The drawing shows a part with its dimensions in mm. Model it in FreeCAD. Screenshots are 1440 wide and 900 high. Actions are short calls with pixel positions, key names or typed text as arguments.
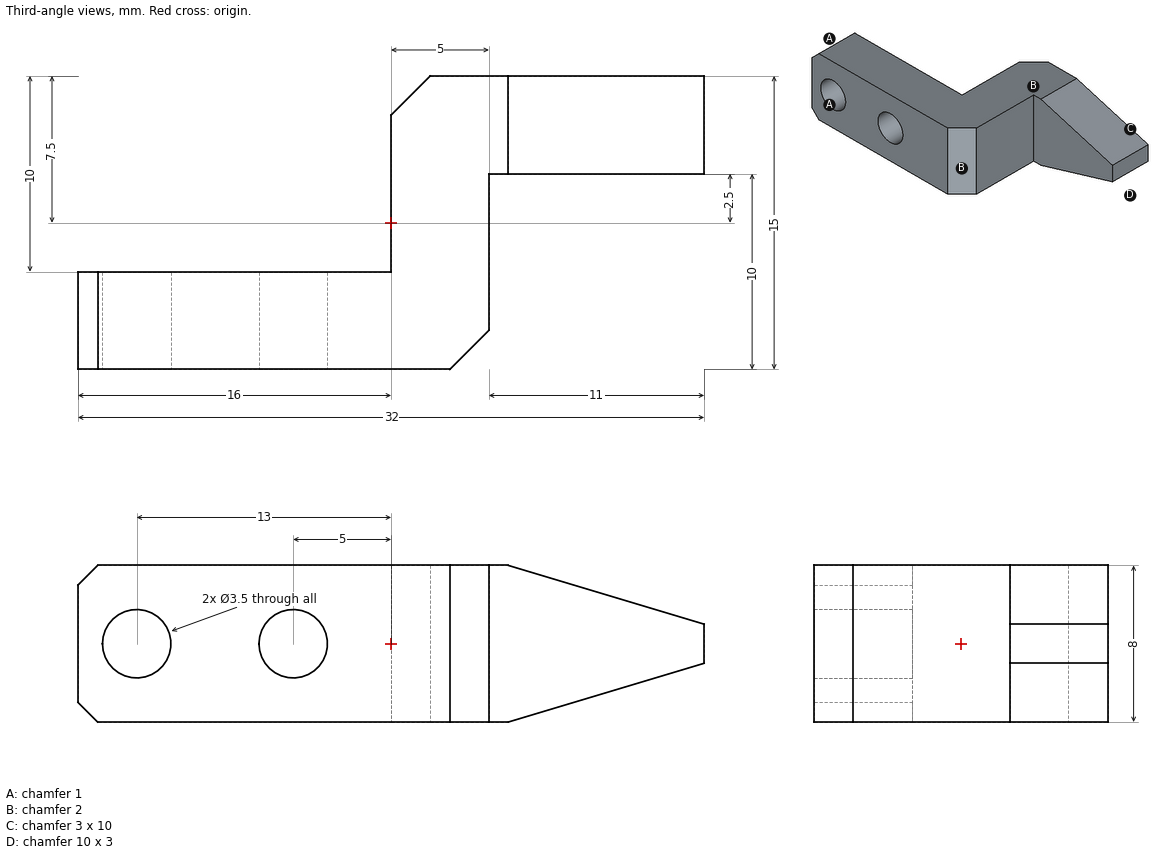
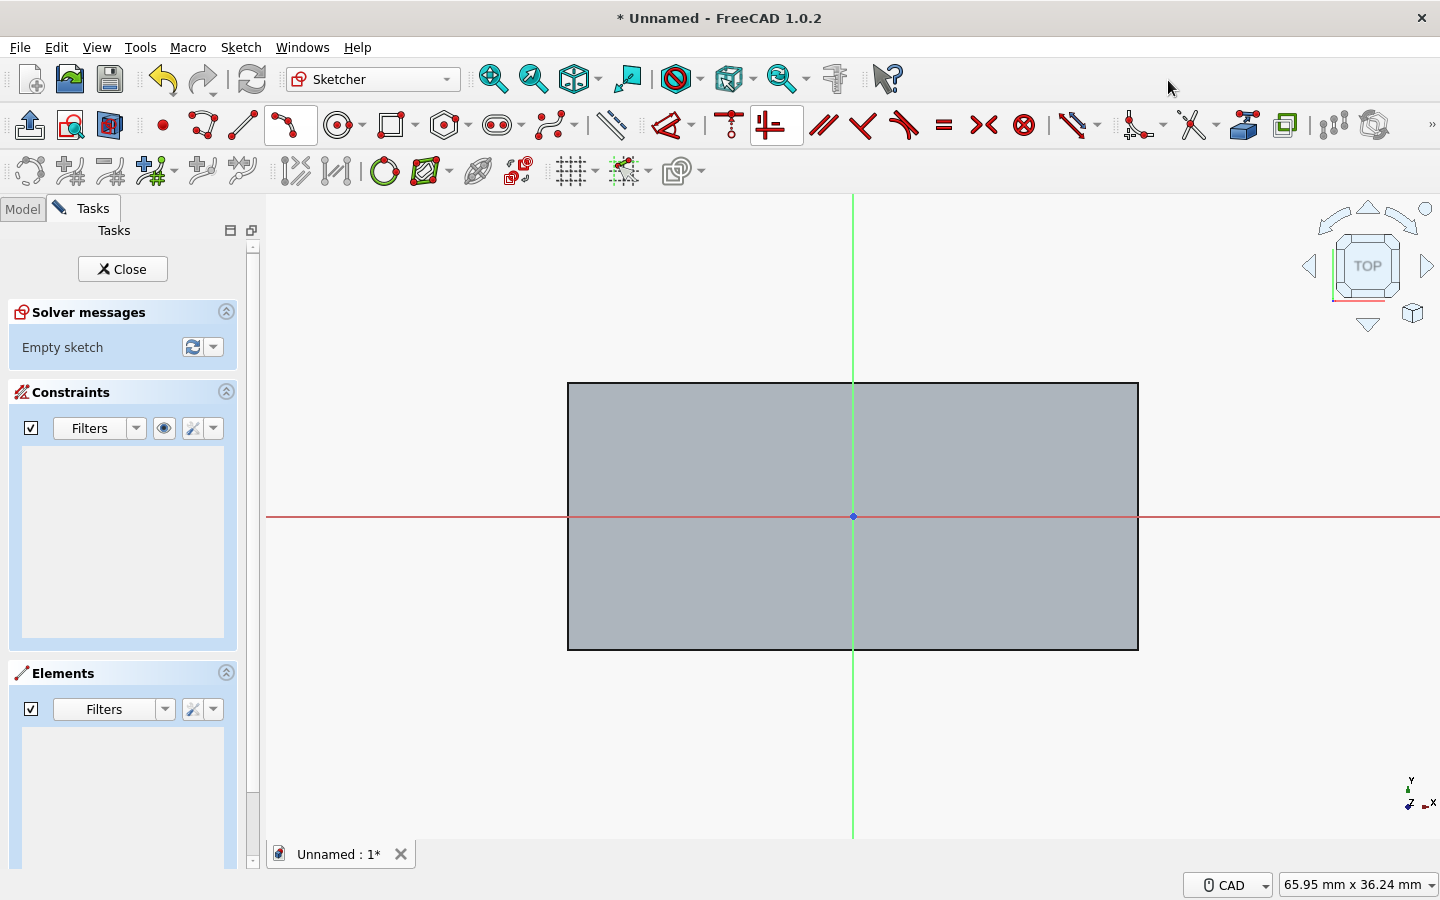
key(g)
key(r)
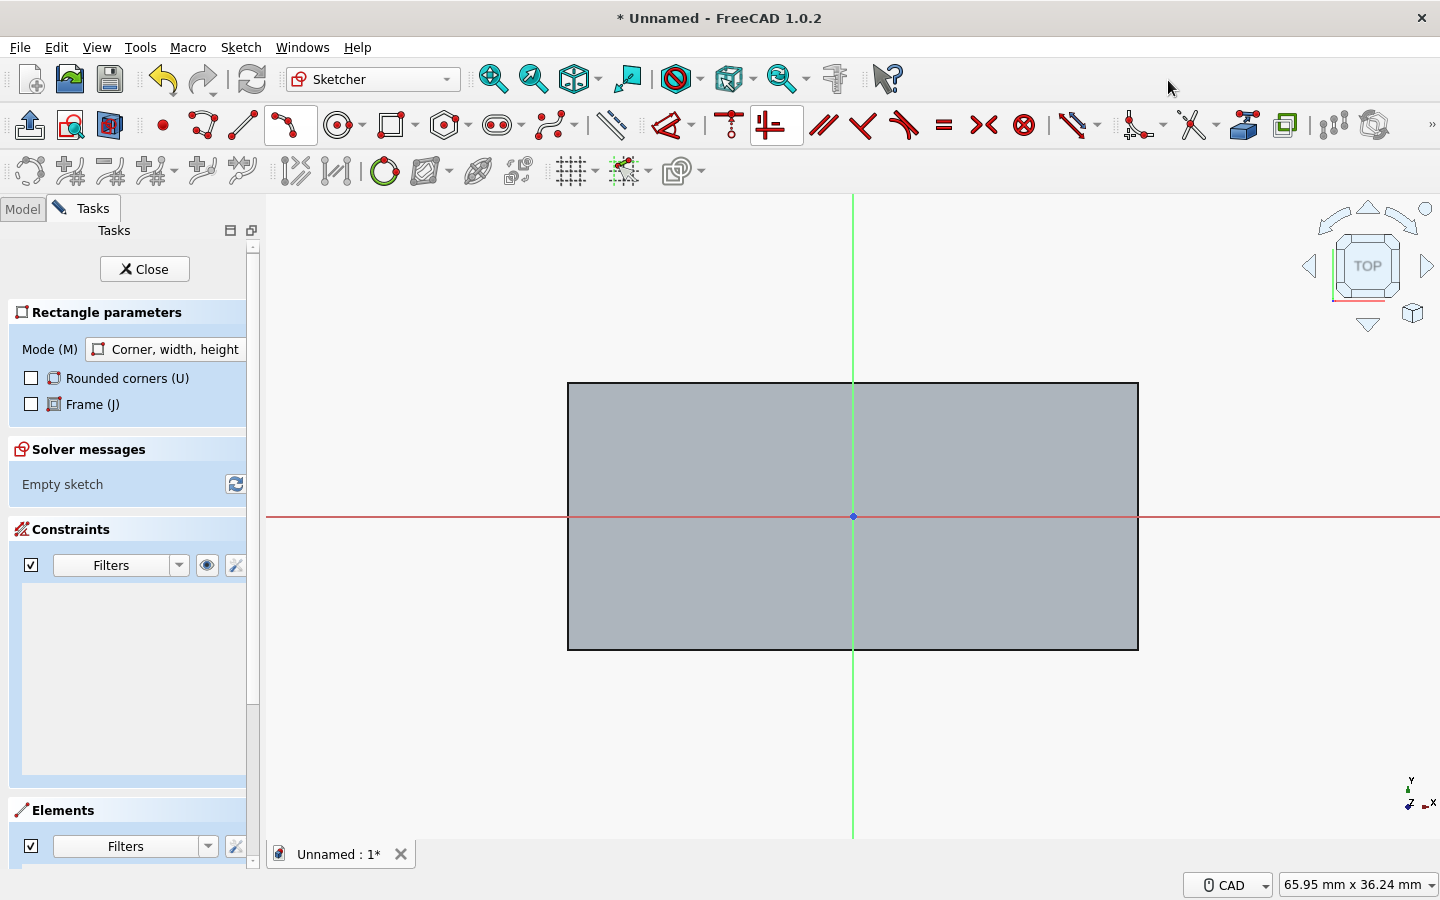
click(568, 383)
click(853, 561)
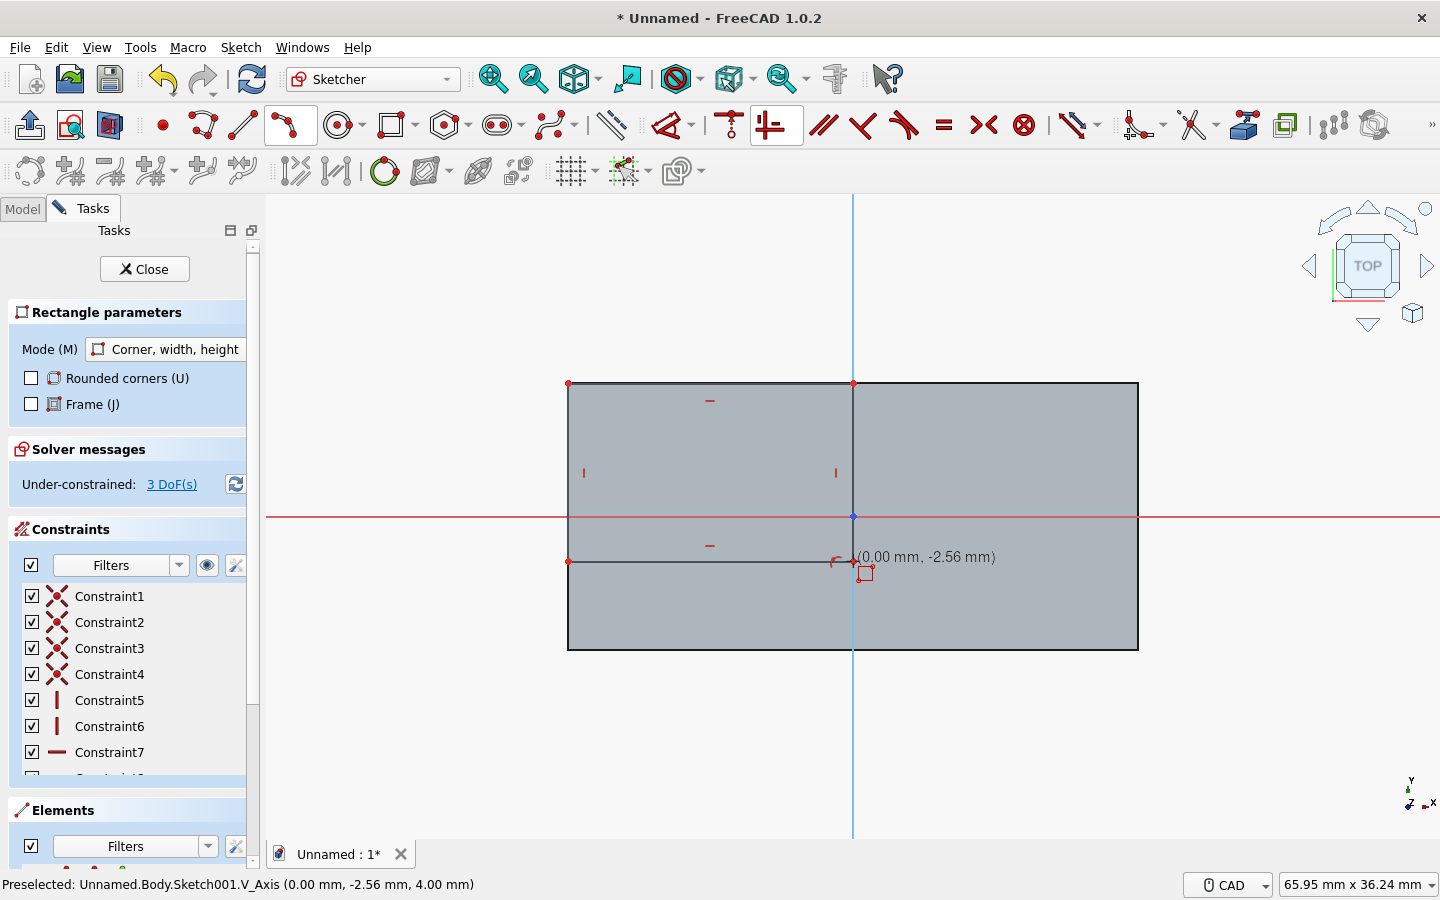
click(942, 472)
move(1138, 650)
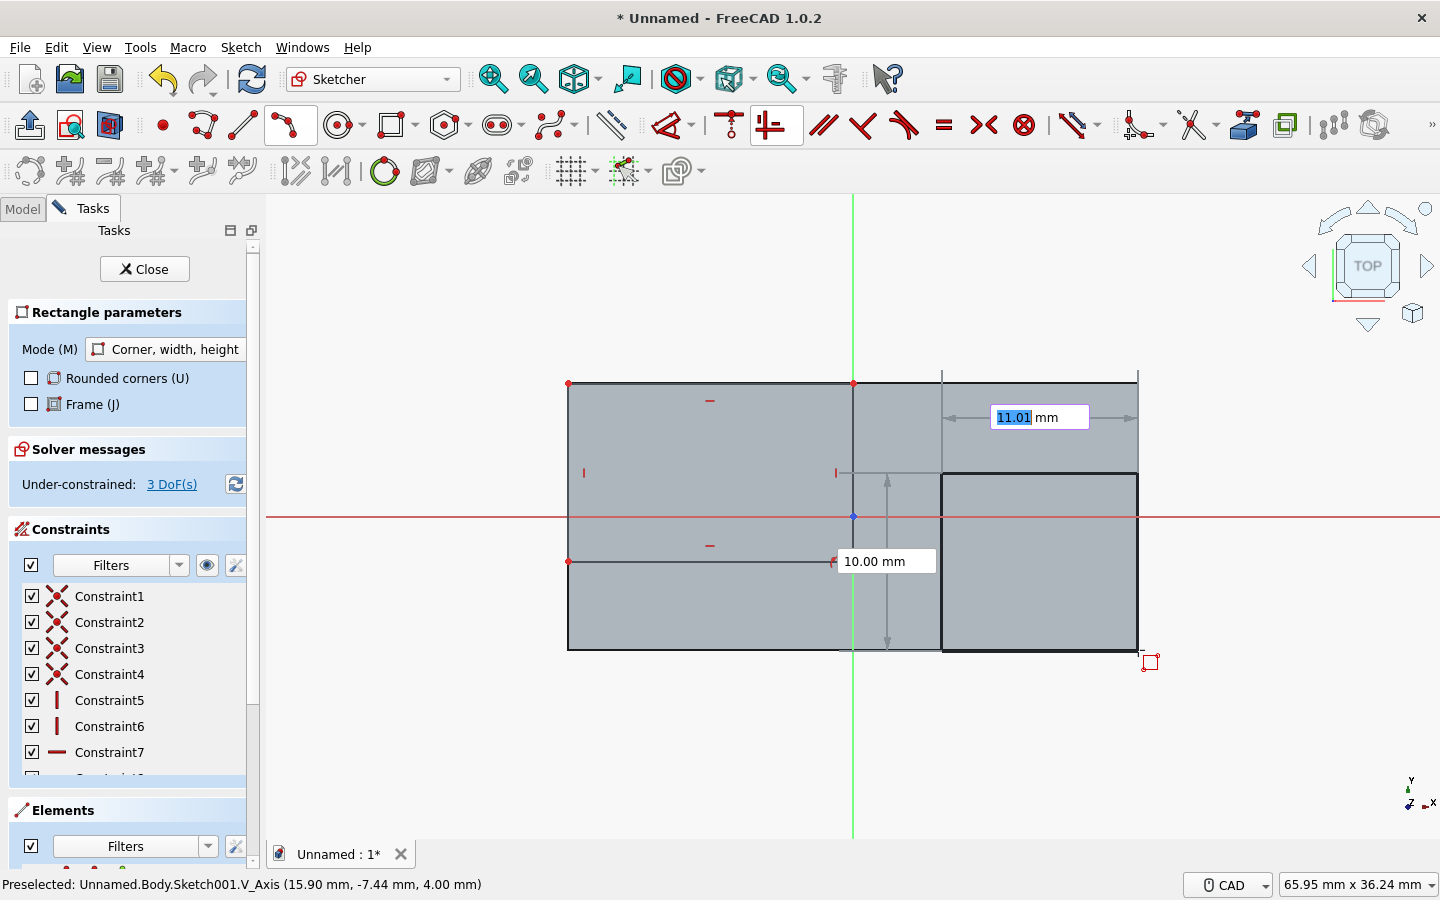
text(11)
key(Tab)
text(10)
key(Return)
key(Escape)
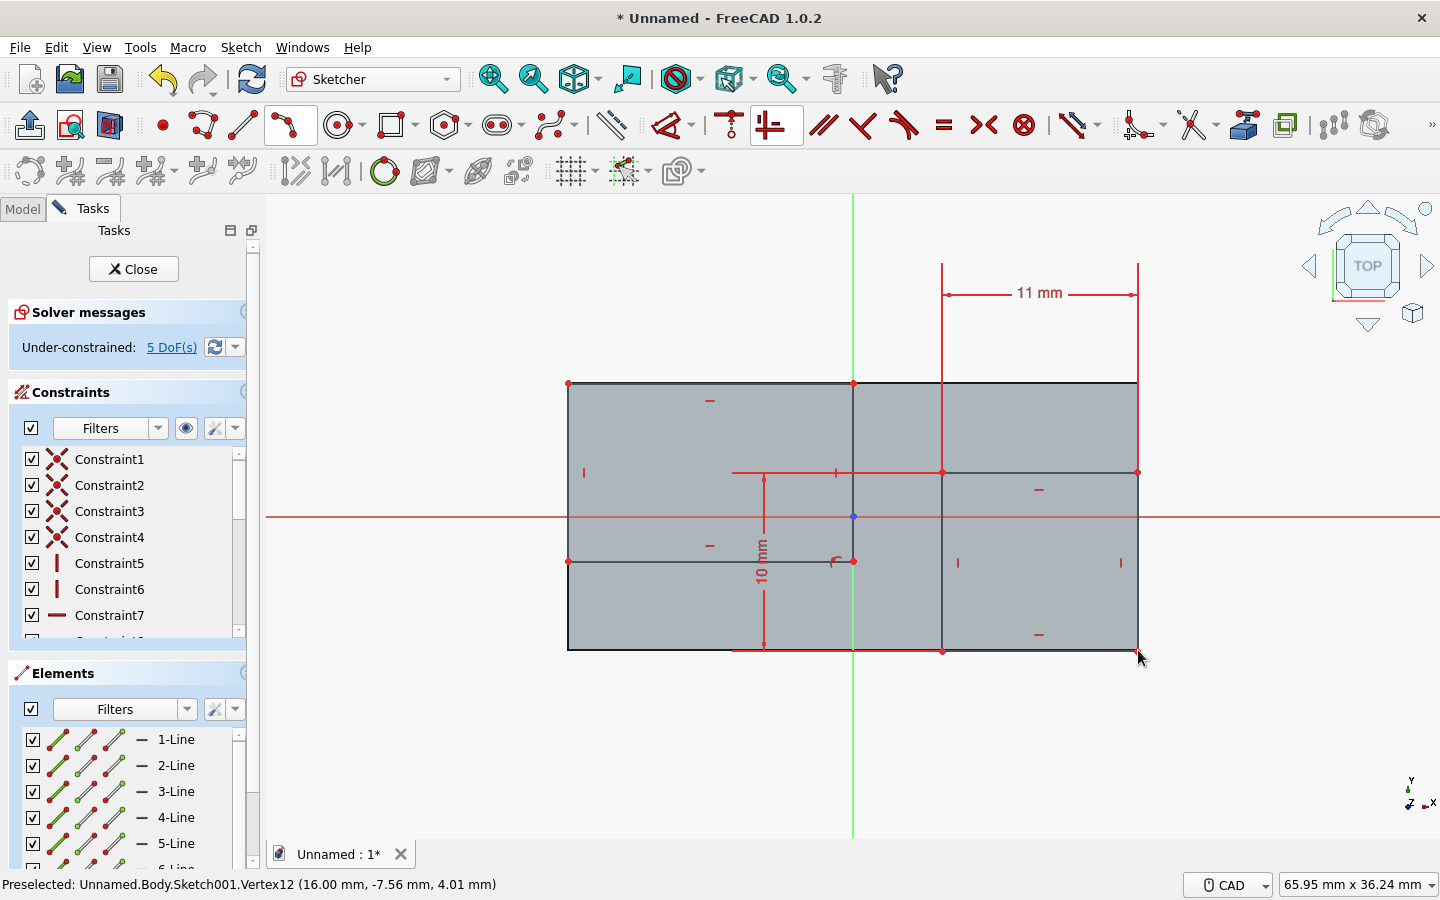
key(d)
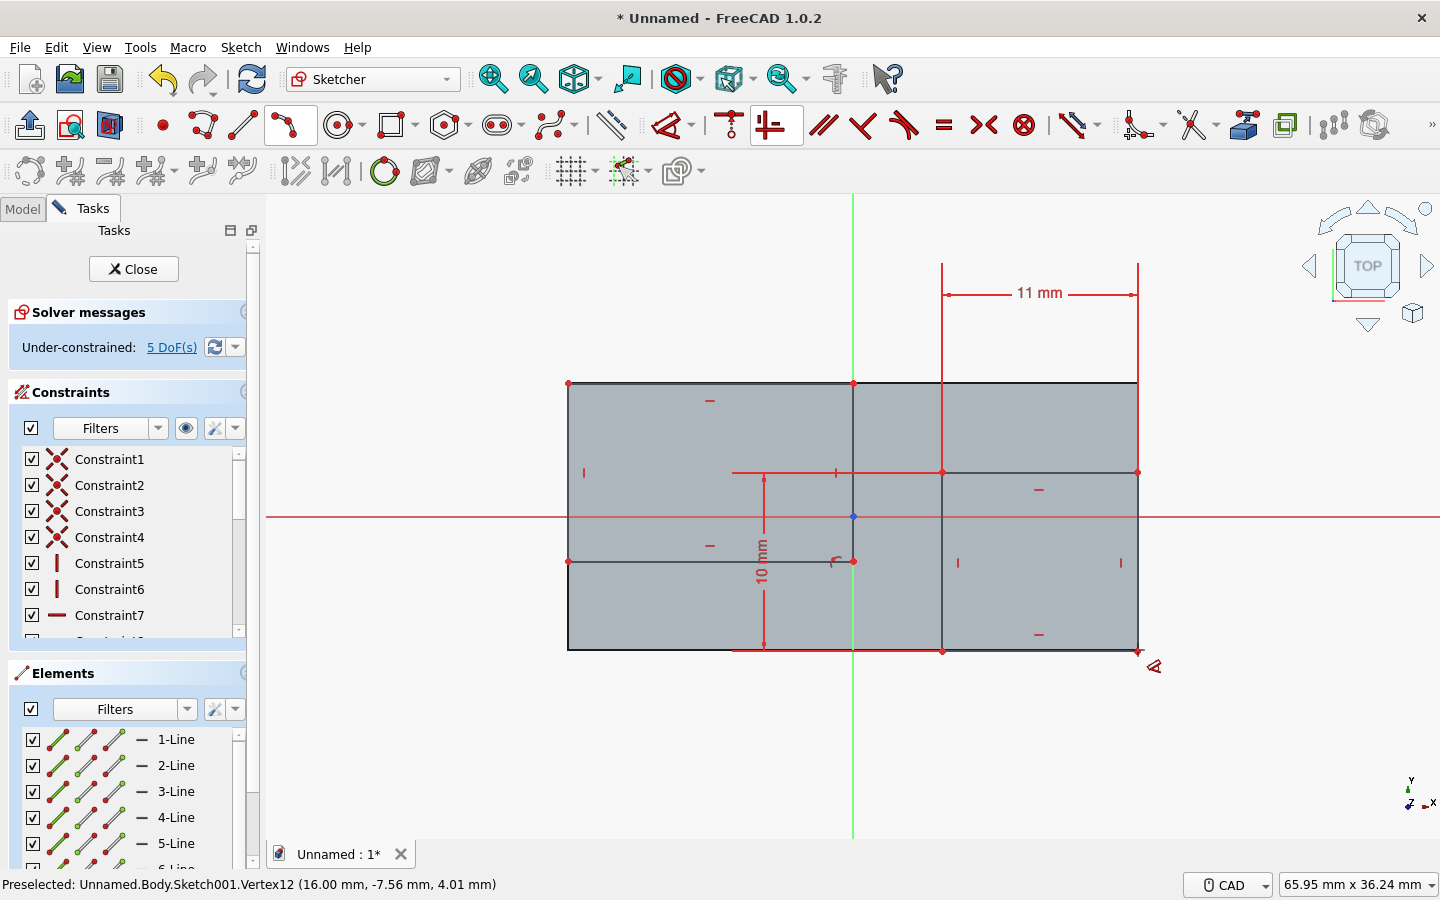
click(568, 437)
click(534, 473)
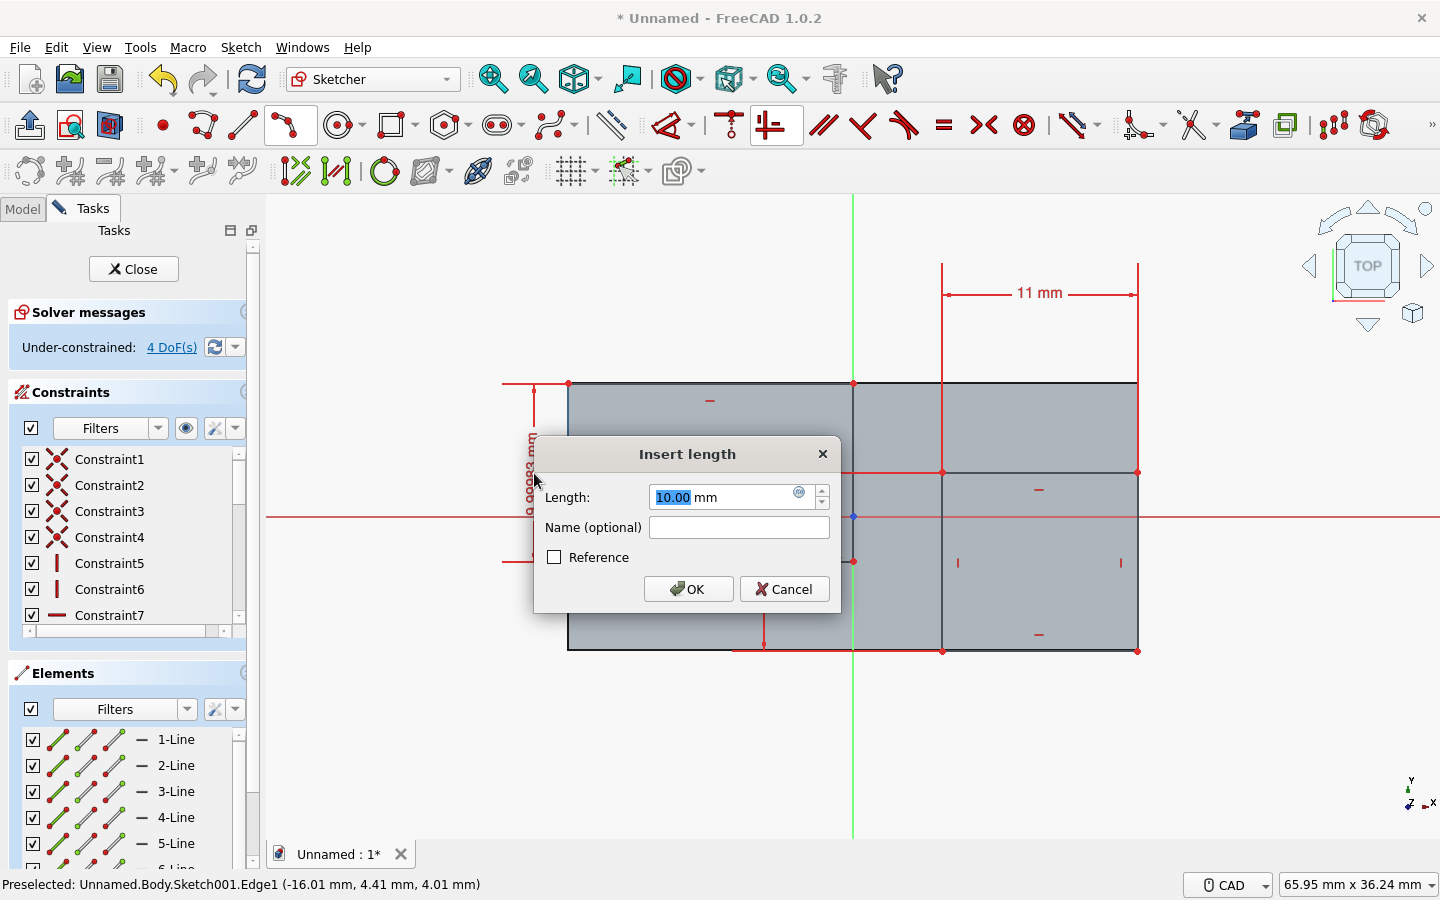
text(10)
key(Return)